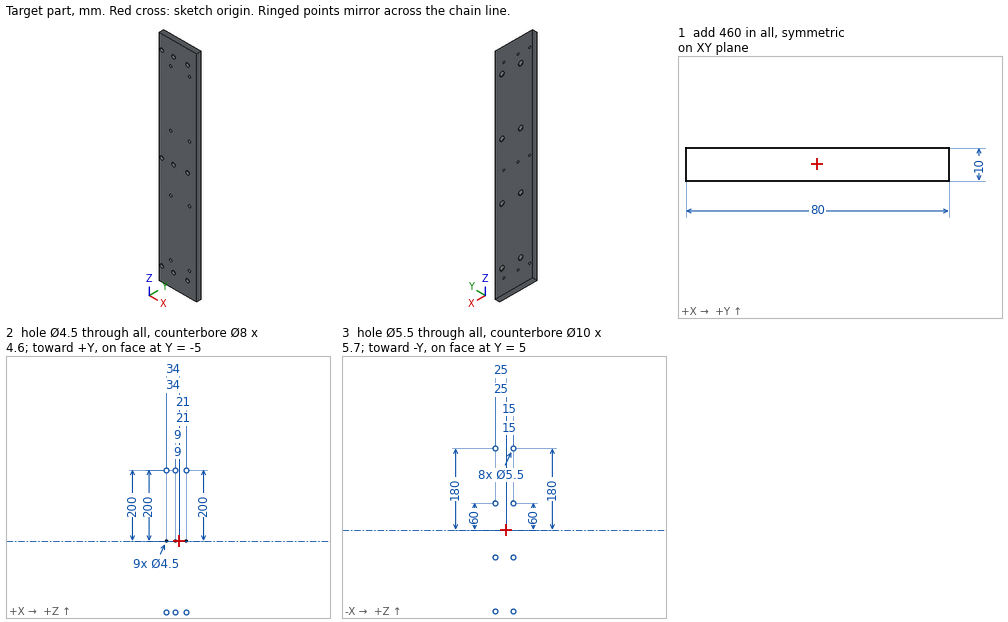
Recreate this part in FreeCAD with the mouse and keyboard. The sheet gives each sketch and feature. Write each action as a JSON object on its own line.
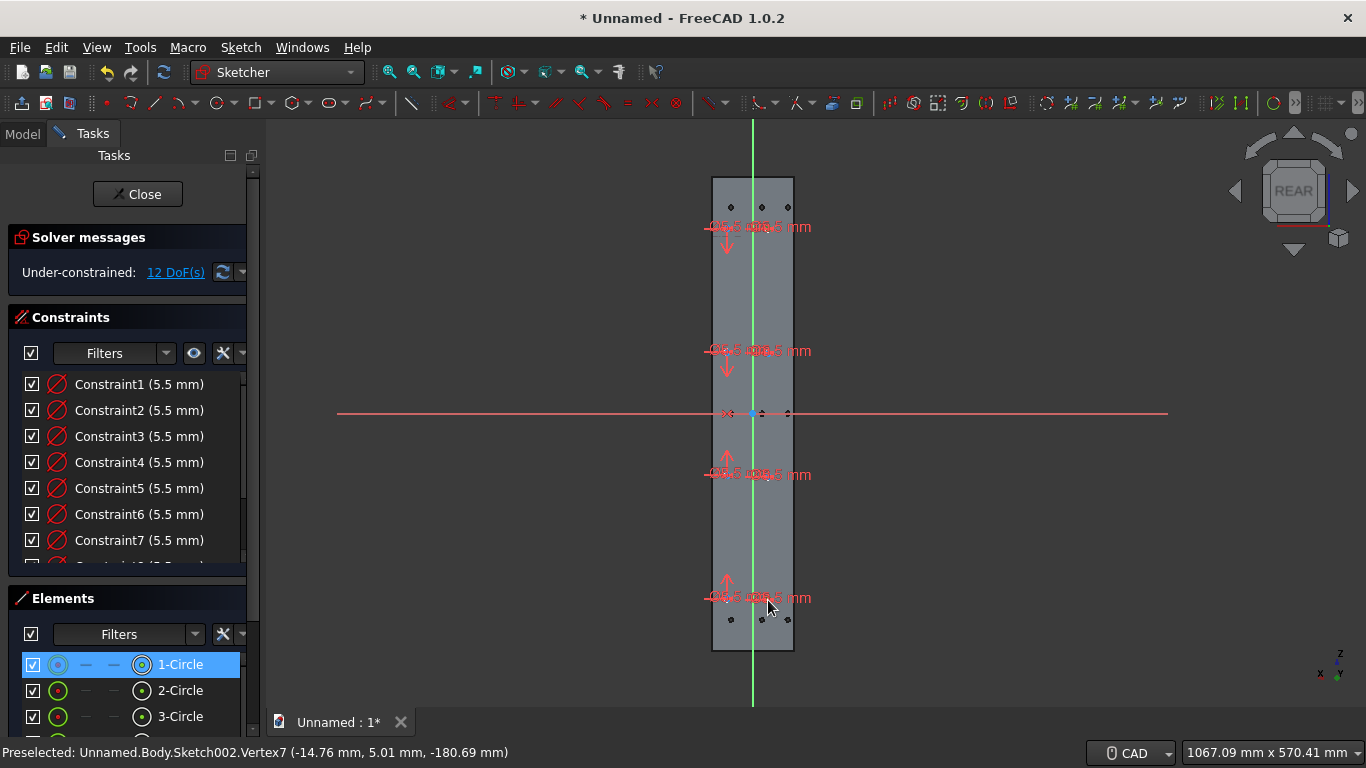
{"action": "left_click", "coordinate": [359, 414]}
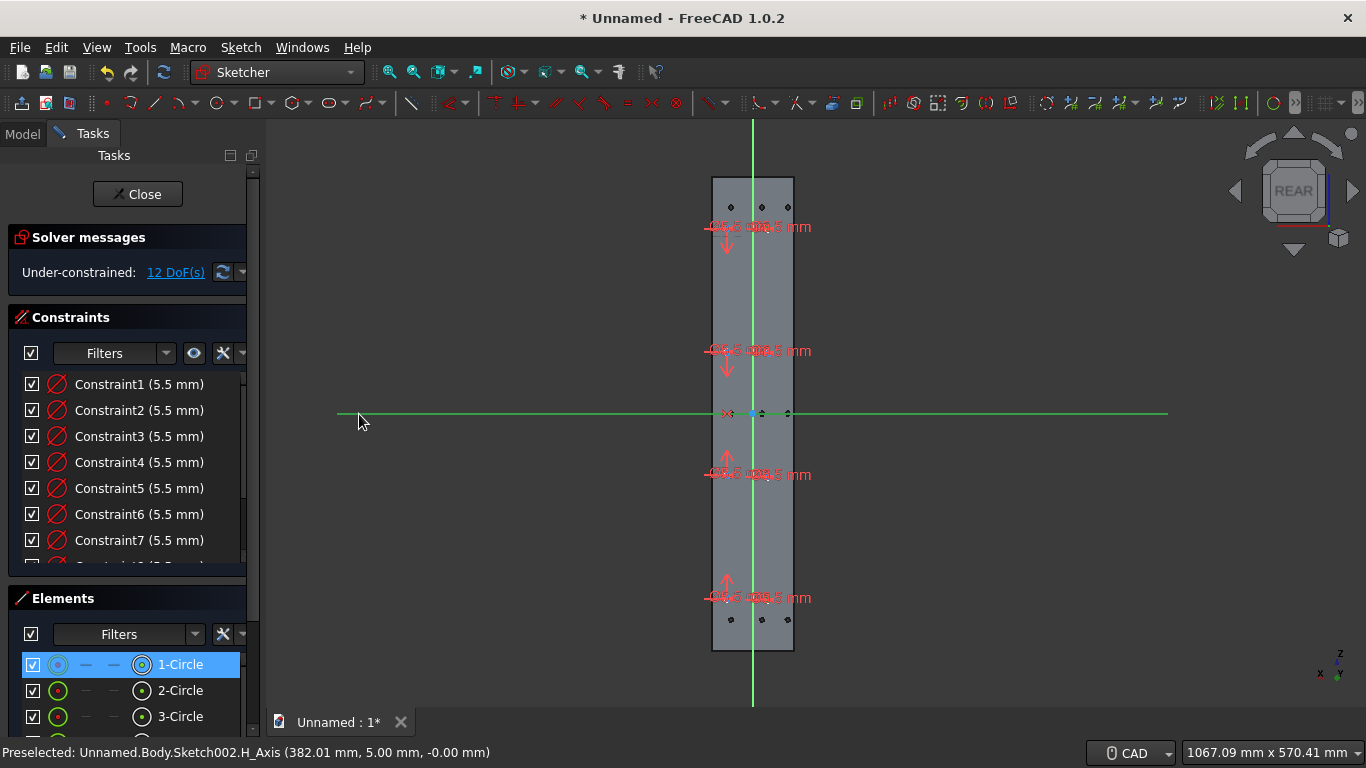
{"action": "key", "text": "s"}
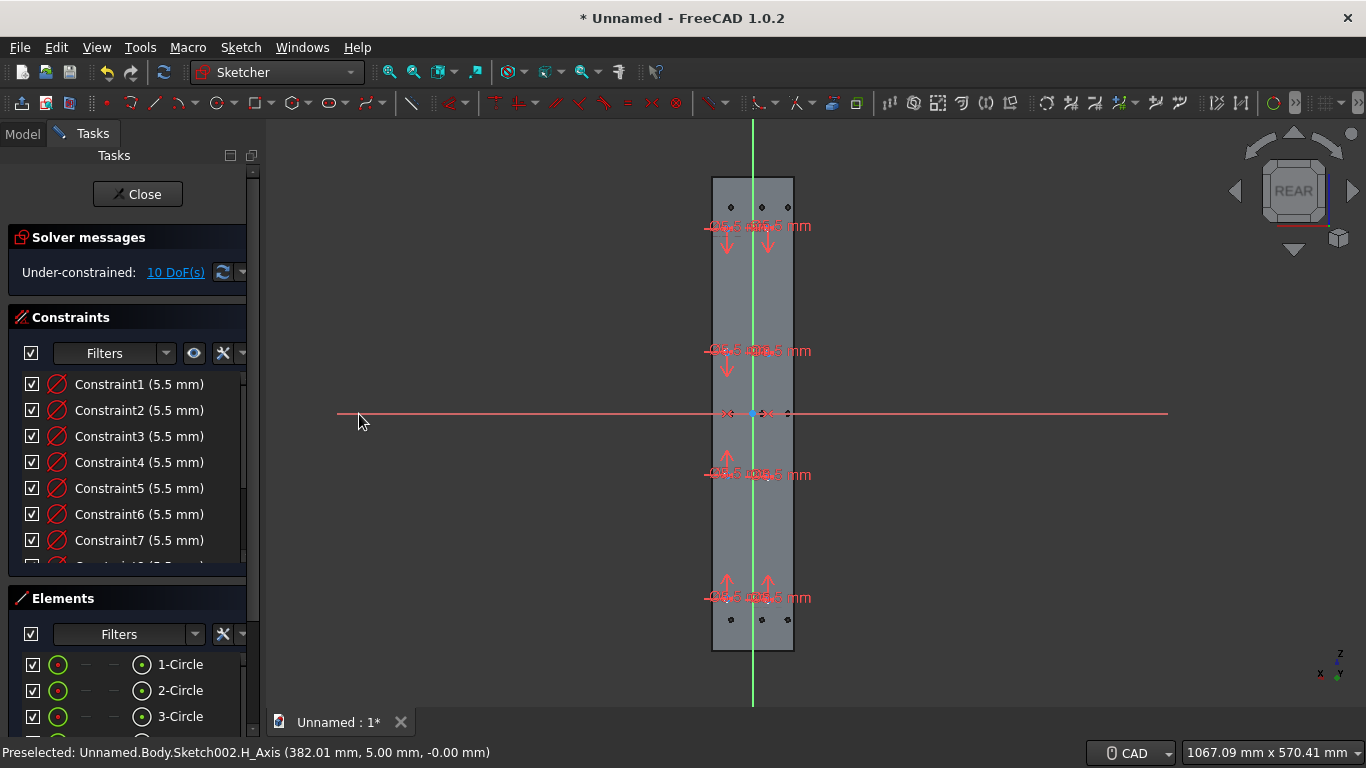
{"action": "left_click", "coordinate": [768, 353]}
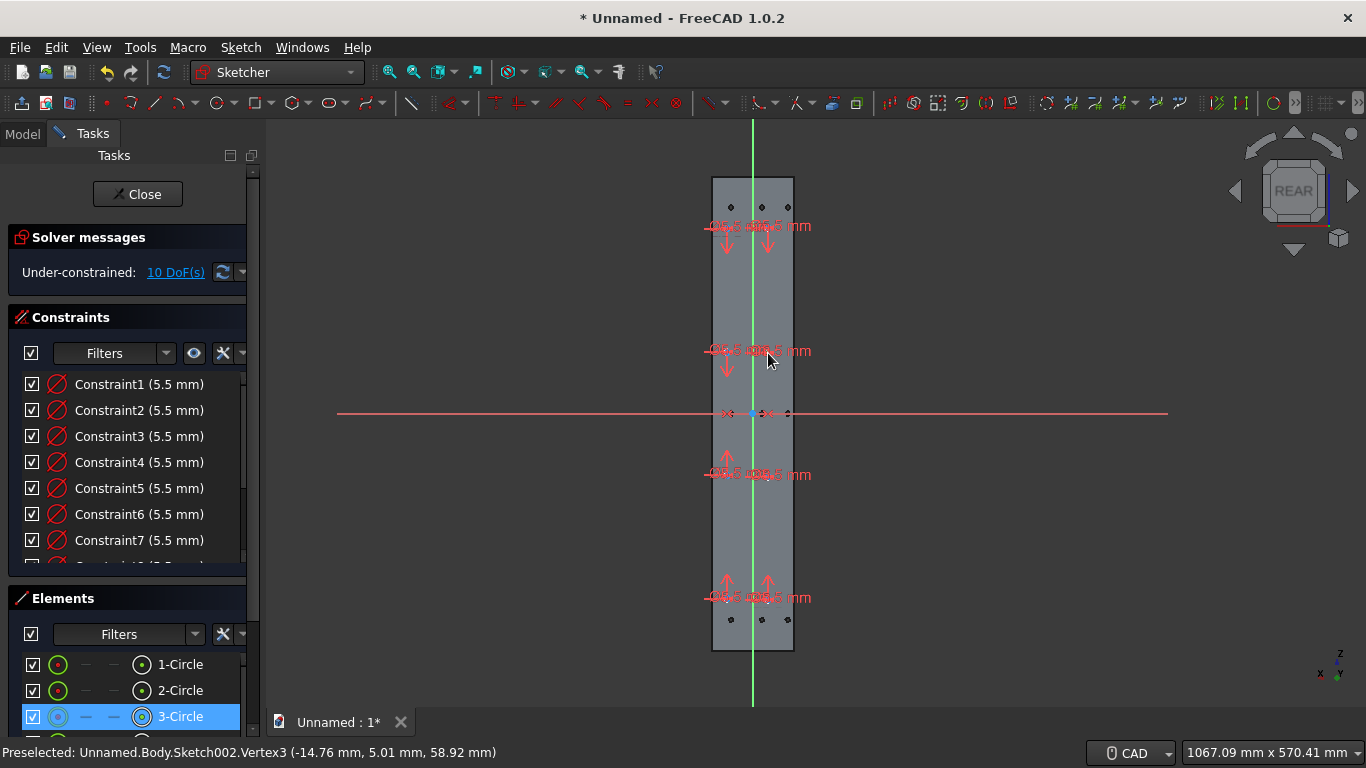
{"action": "left_click", "coordinate": [768, 477]}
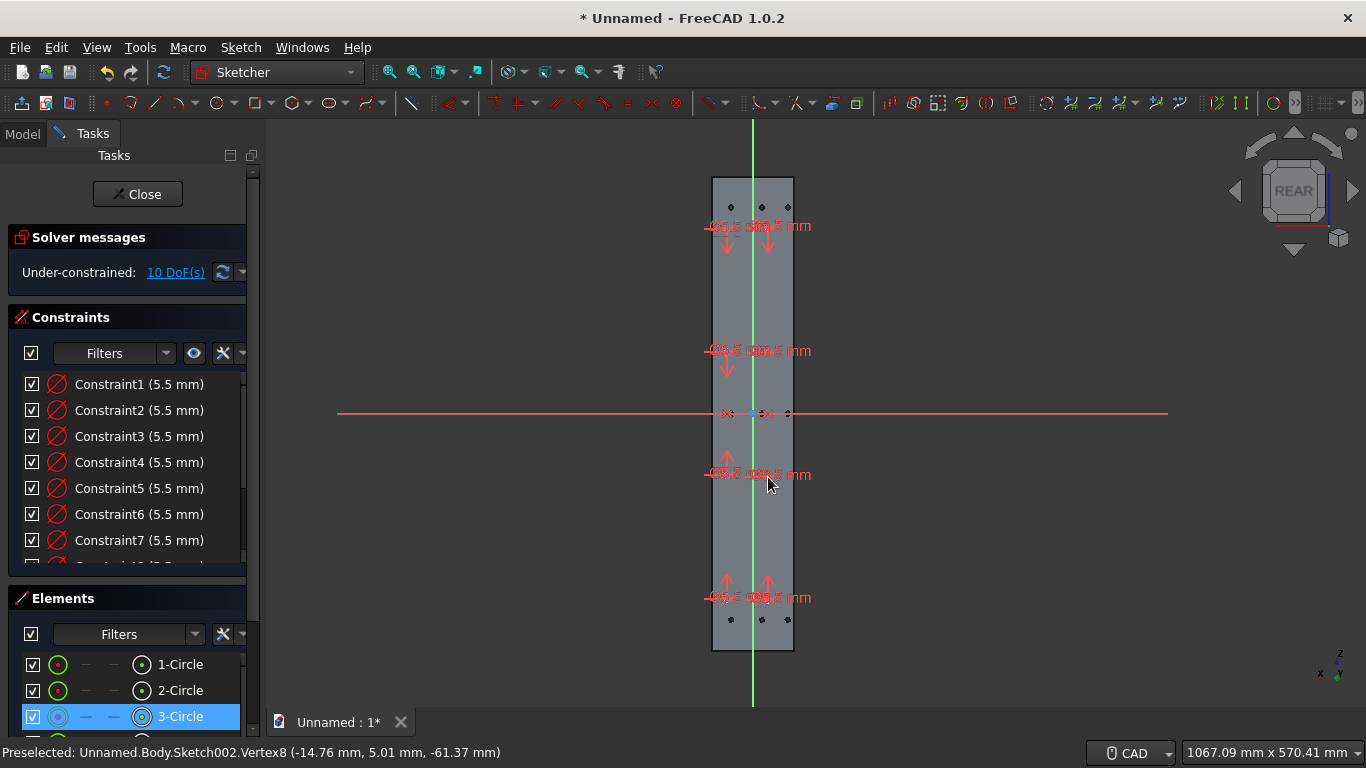
{"action": "left_click", "coordinate": [359, 414]}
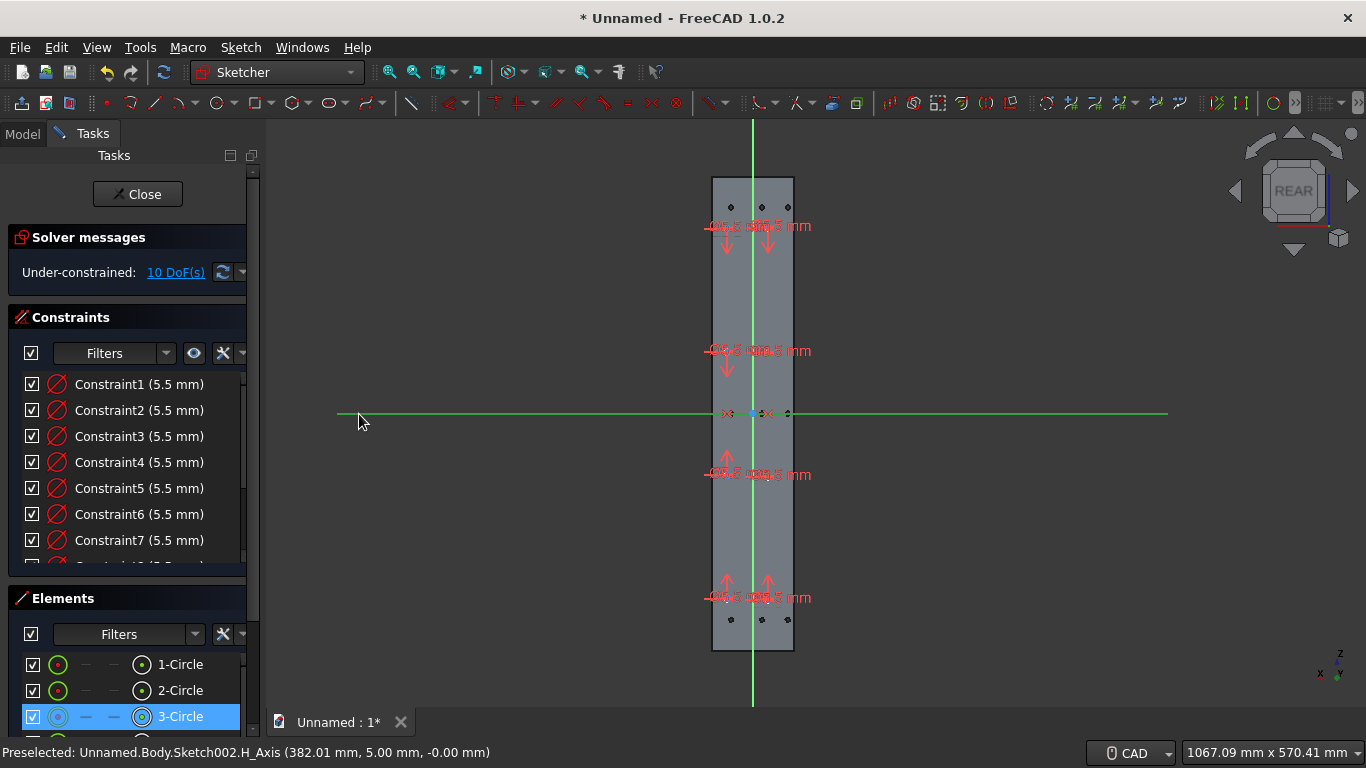
{"action": "key", "text": "s"}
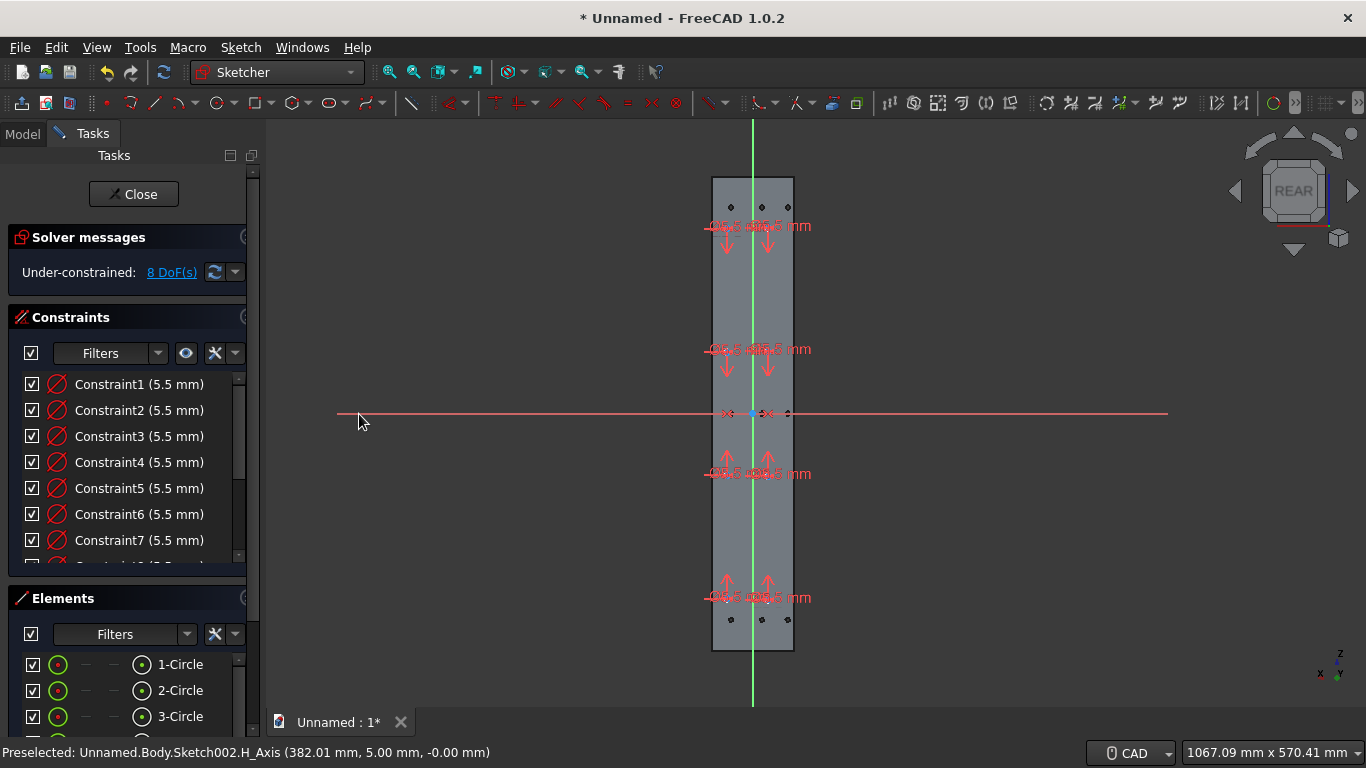
{"action": "key", "text": "d"}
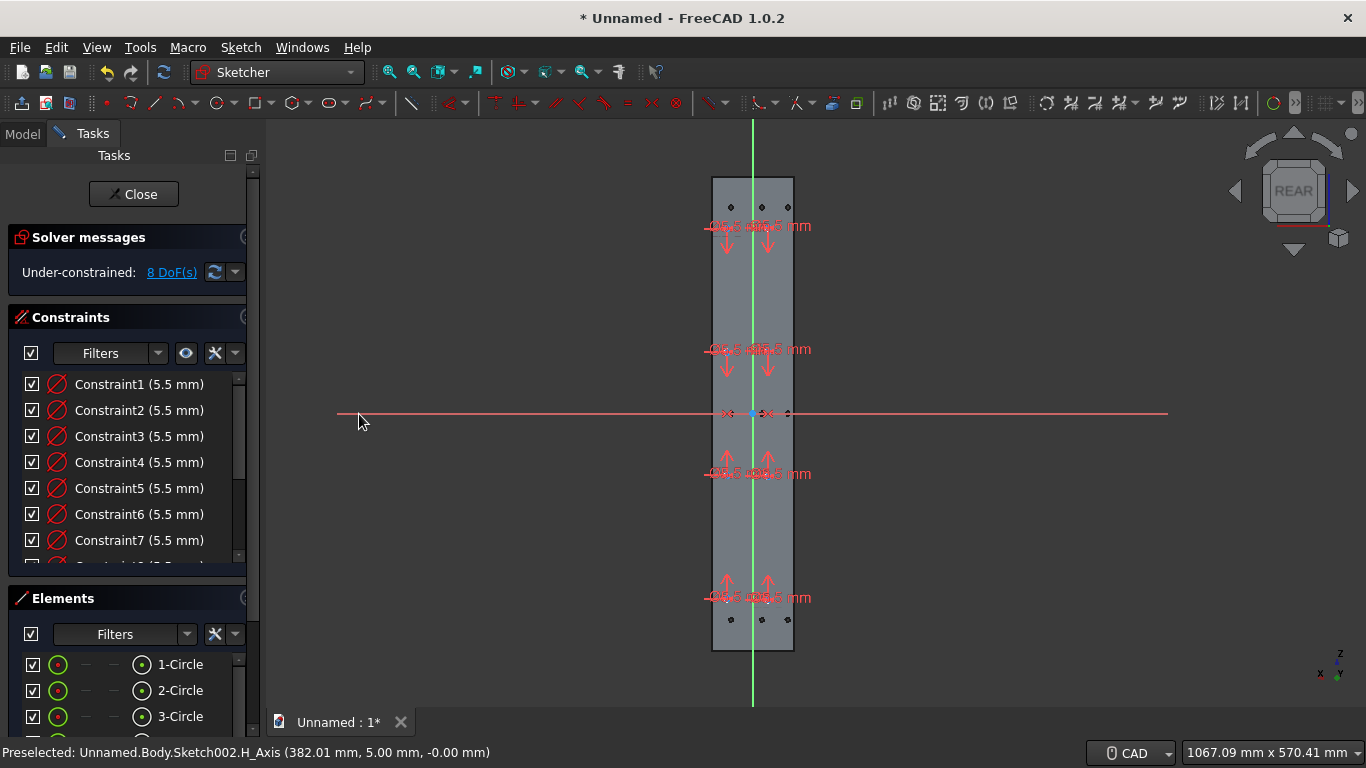
{"action": "scroll", "coordinate": [768, 228], "scroll_direction": "up", "scroll_amount": 5}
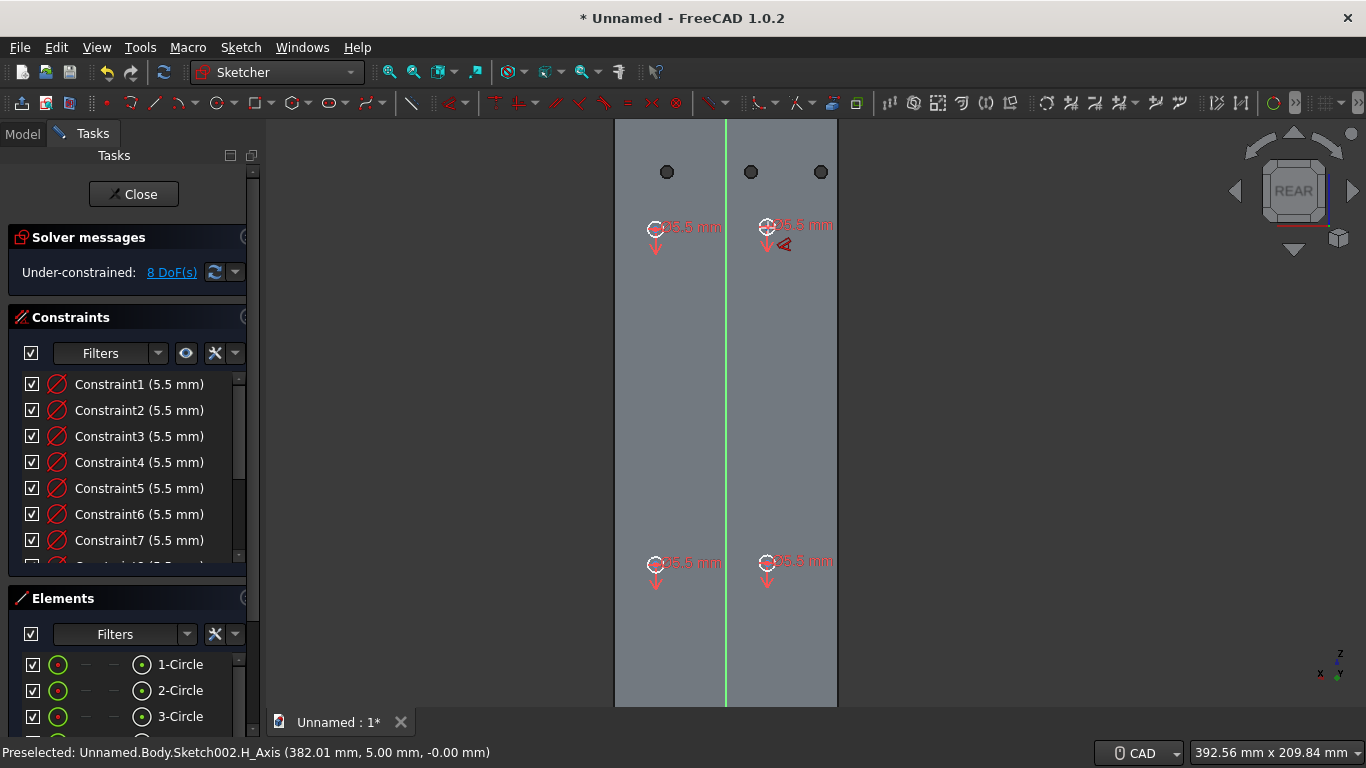
{"action": "left_click", "coordinate": [767, 227]}
{"action": "left_click", "coordinate": [747, 193]}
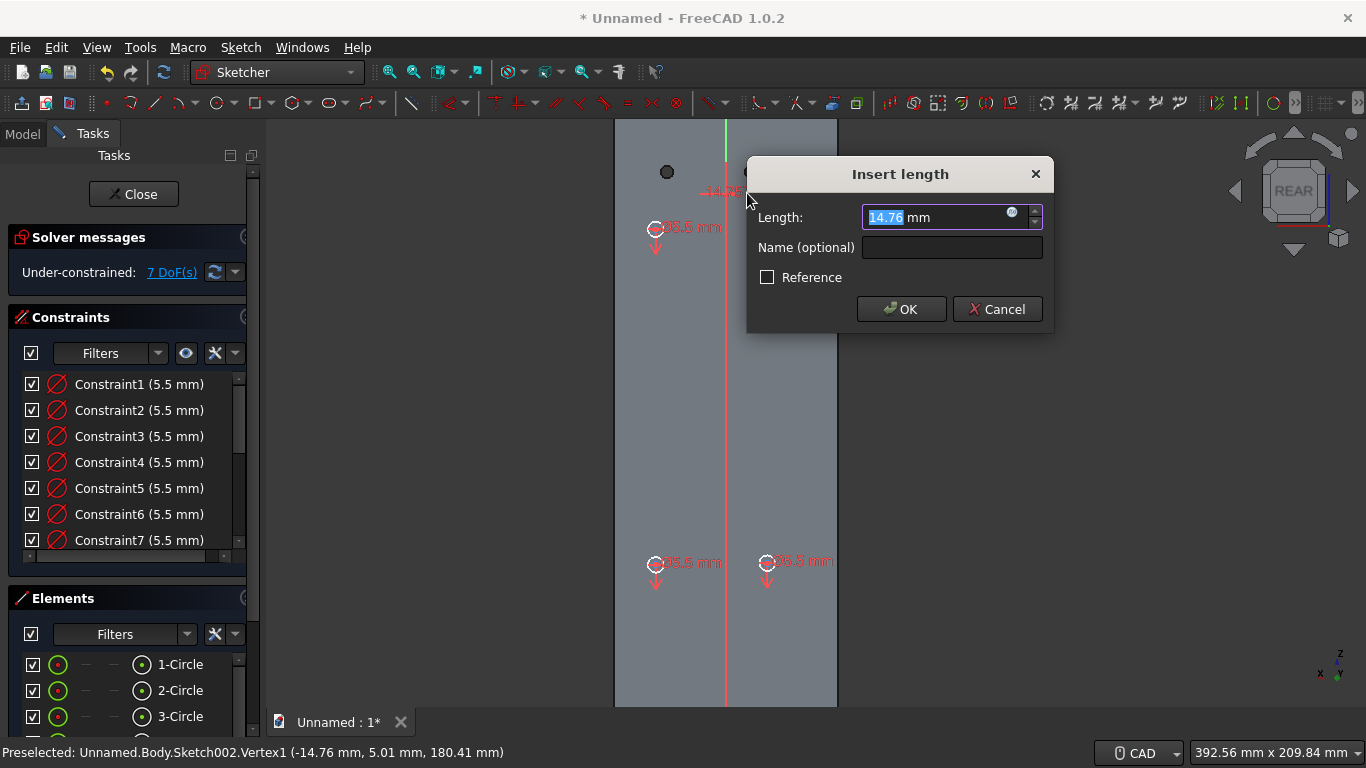
{"action": "type", "text": "15"}
{"action": "key", "text": "Return"}